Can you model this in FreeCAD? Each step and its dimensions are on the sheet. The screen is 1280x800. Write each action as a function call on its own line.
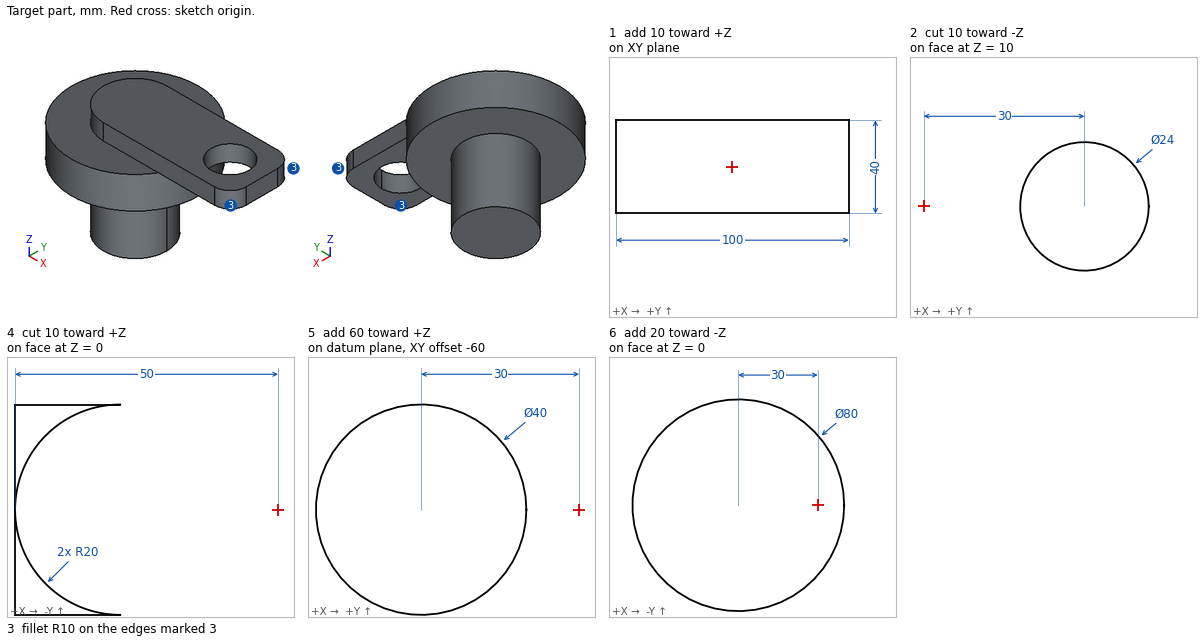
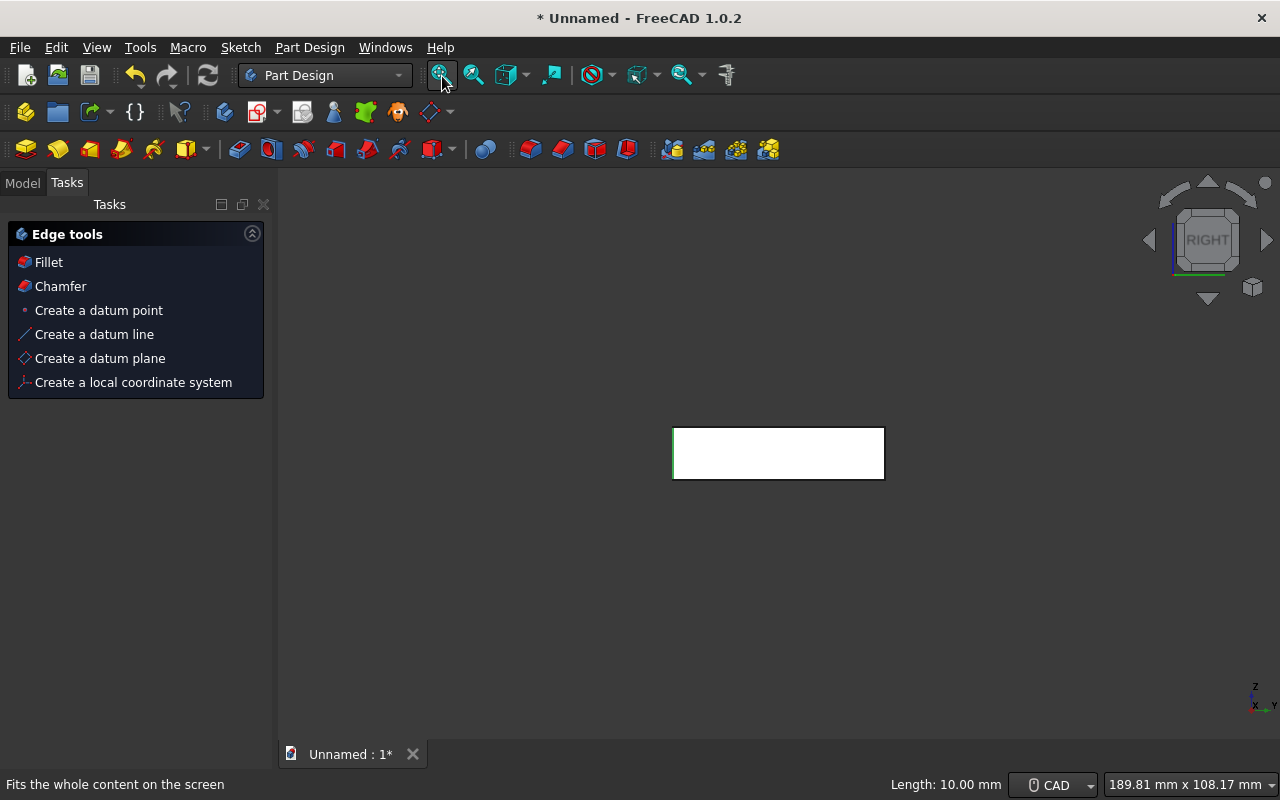
click(885, 452, ctrl)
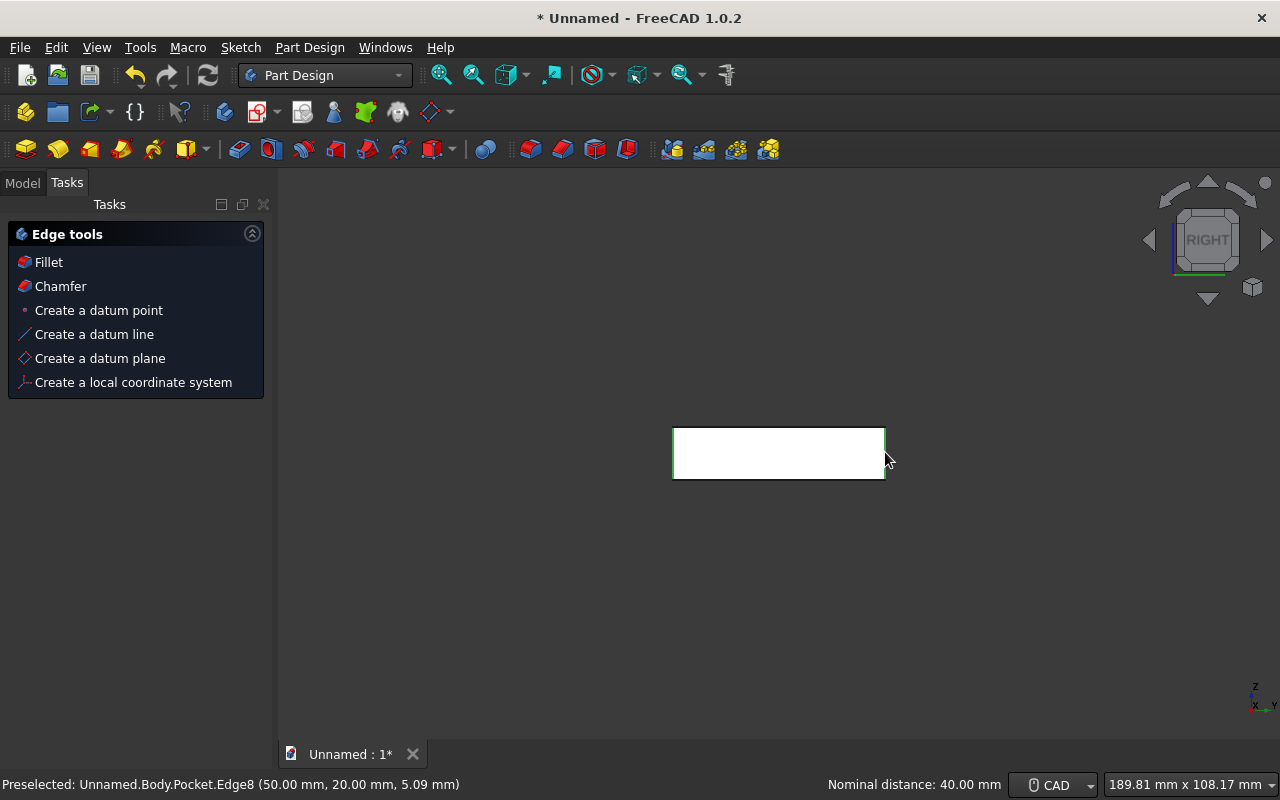
click(532, 150)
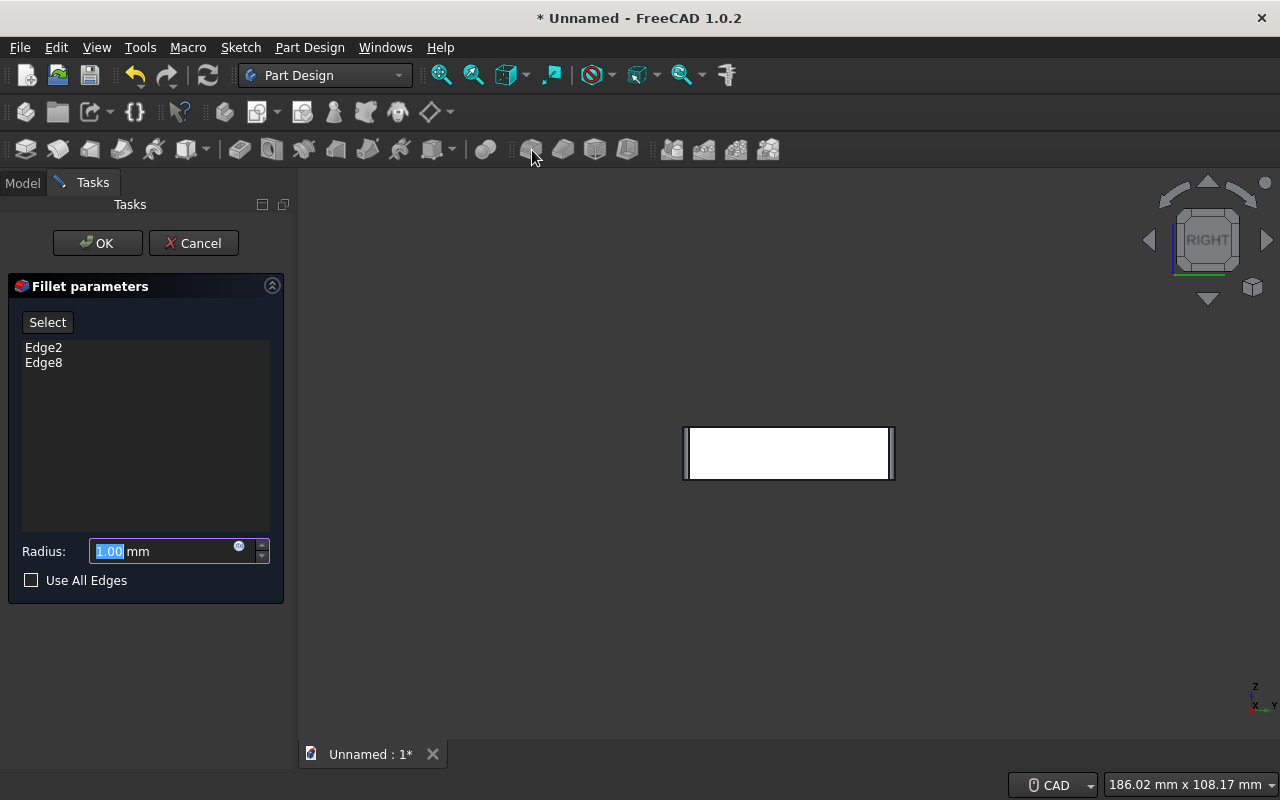
text(10)
key(Tab)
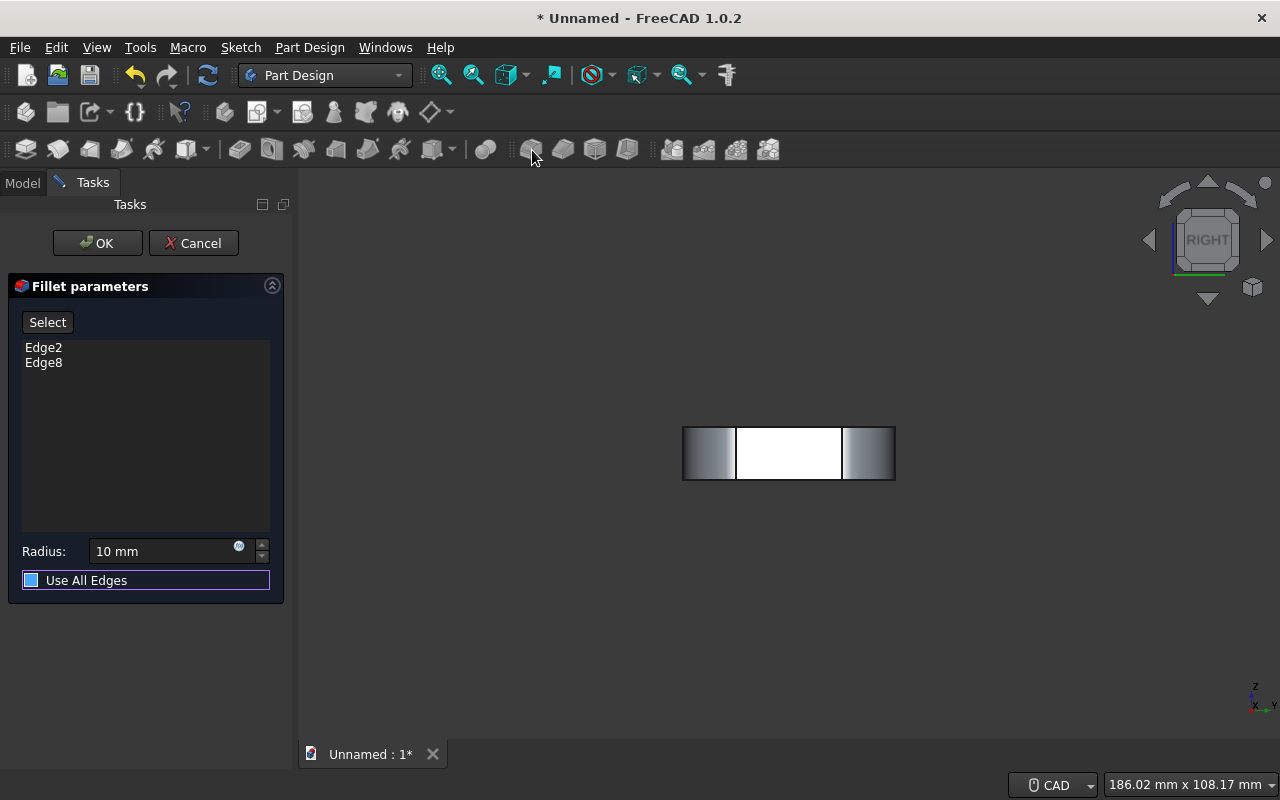
click(98, 243)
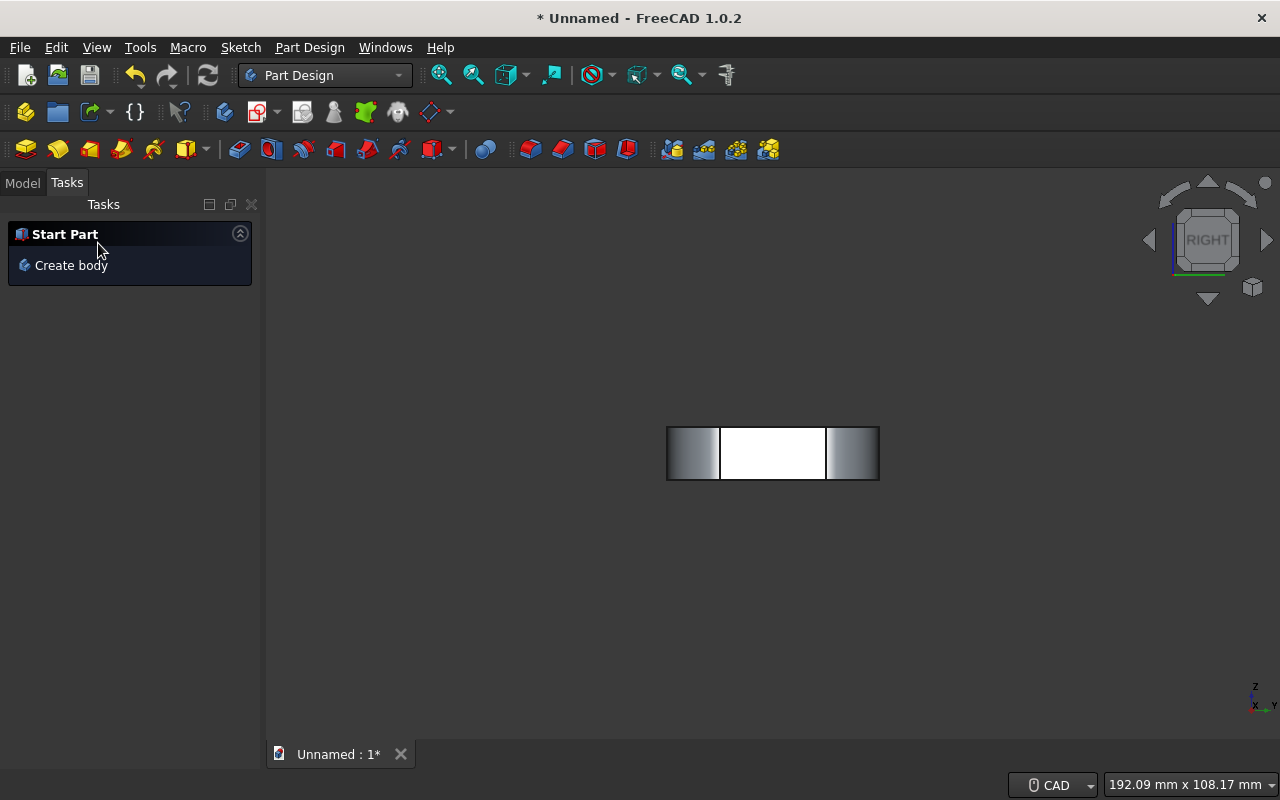
click(442, 76)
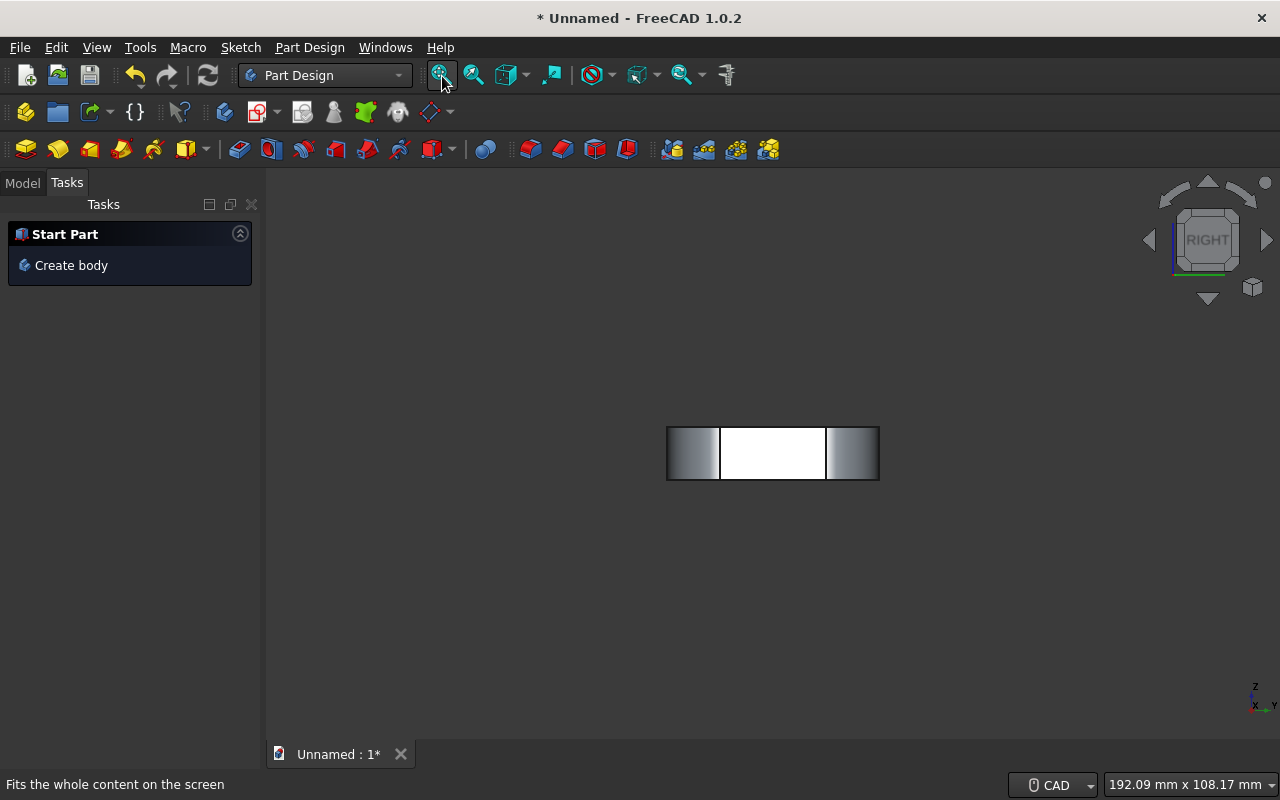
key(5)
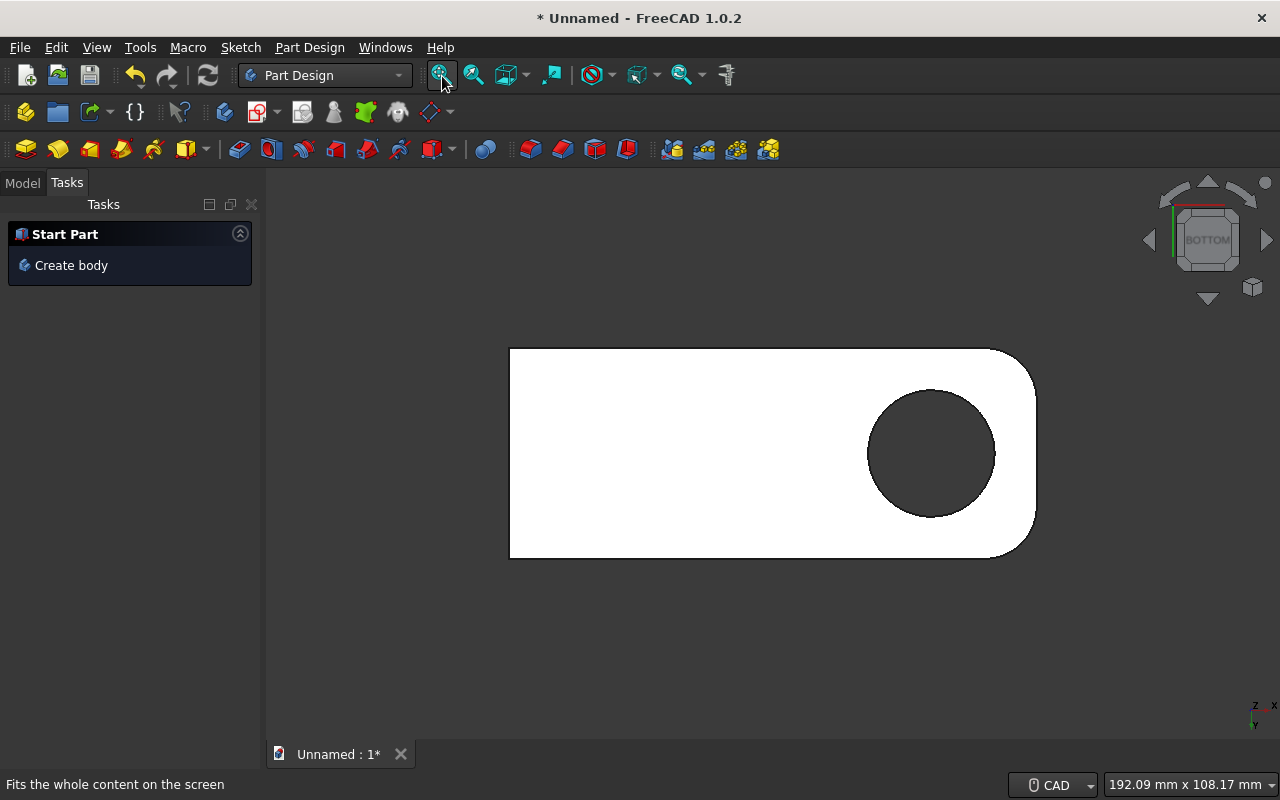
click(698, 452)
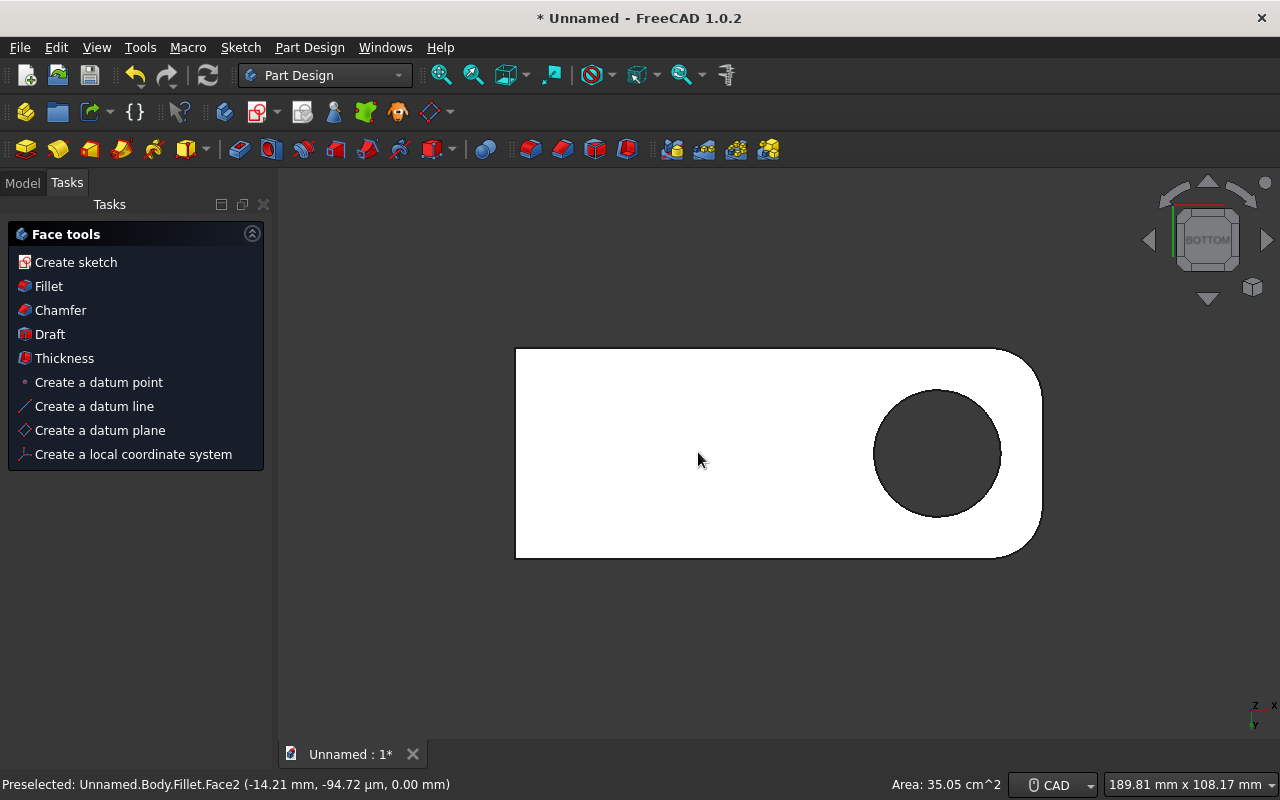
click(258, 112)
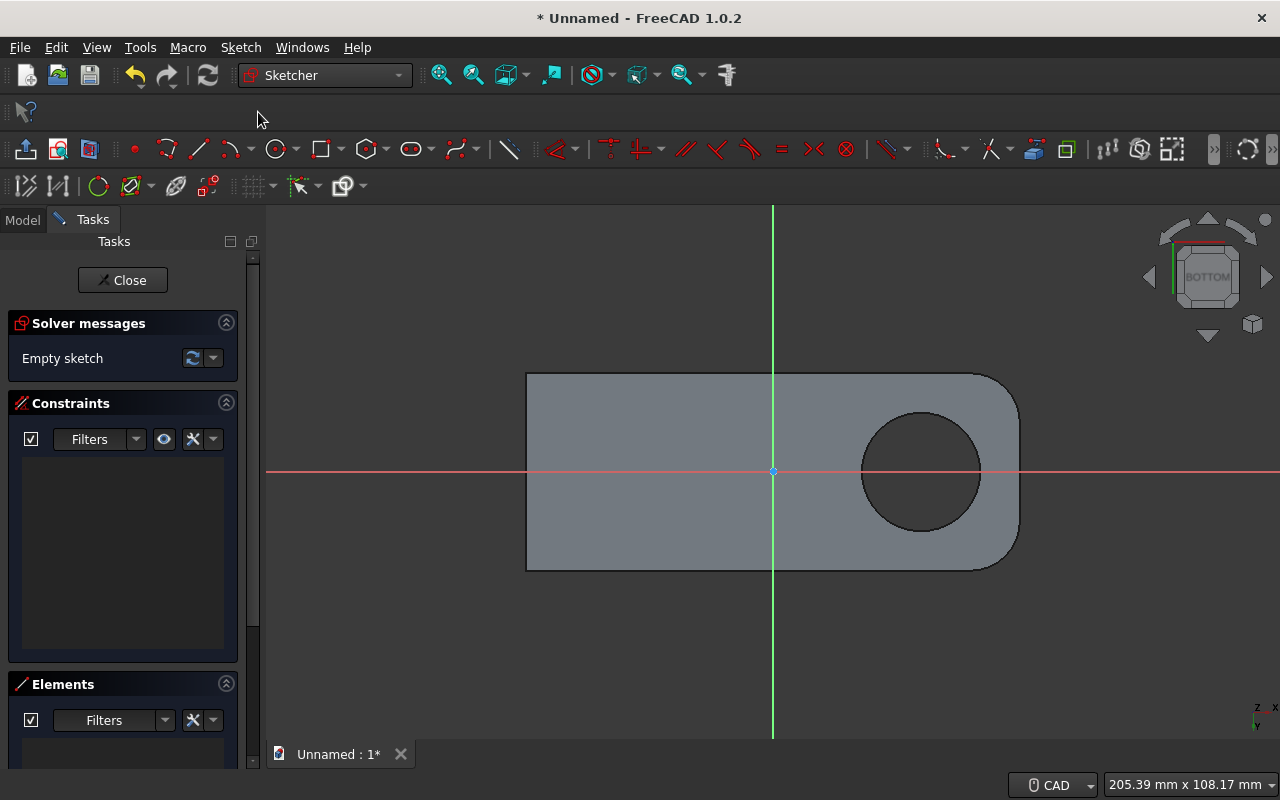
scroll(583, 472, up, 3)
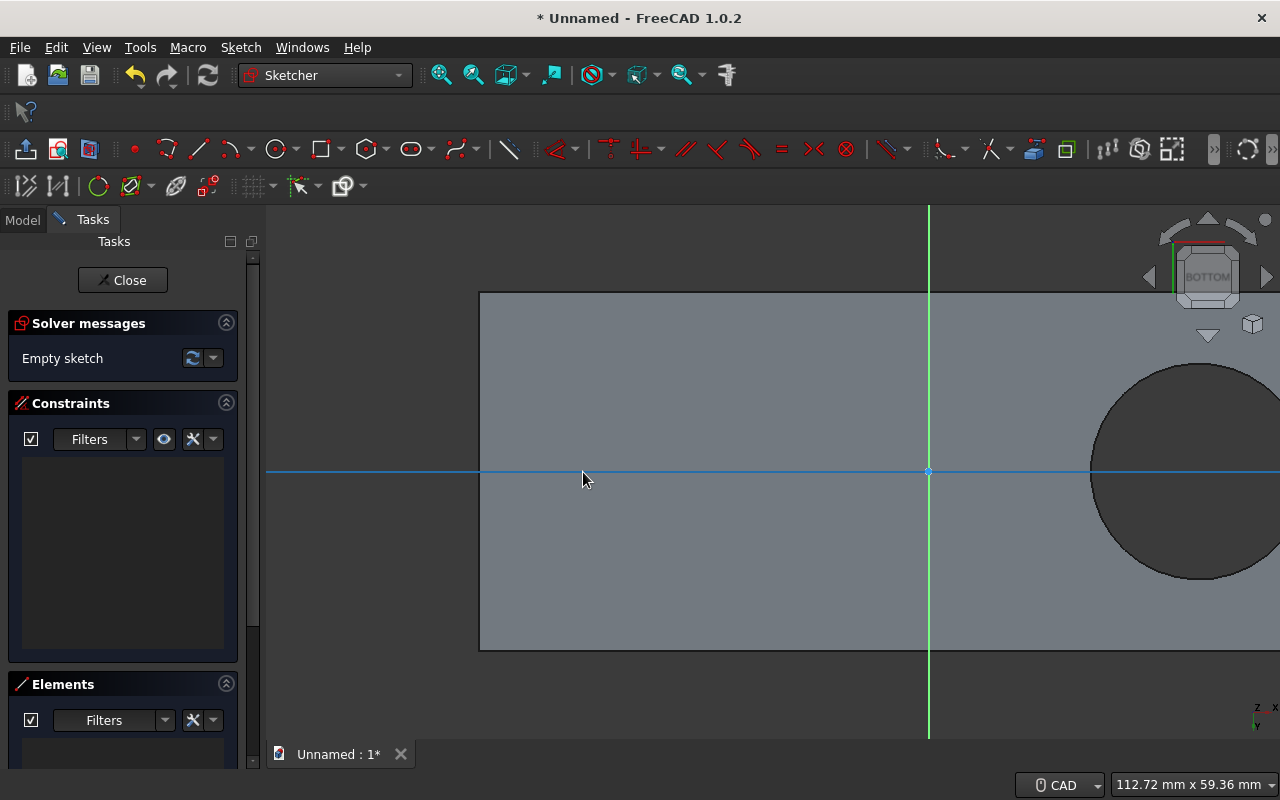
key(g)
key(m)